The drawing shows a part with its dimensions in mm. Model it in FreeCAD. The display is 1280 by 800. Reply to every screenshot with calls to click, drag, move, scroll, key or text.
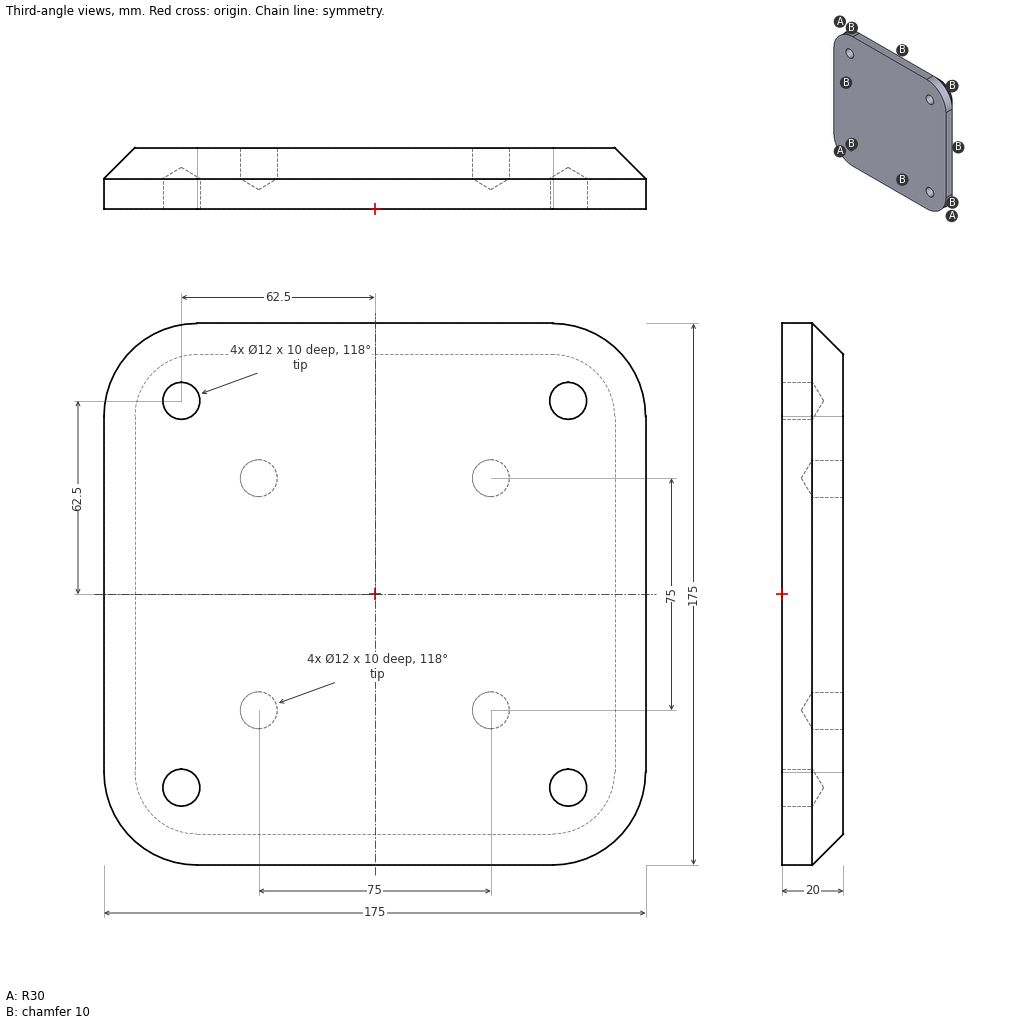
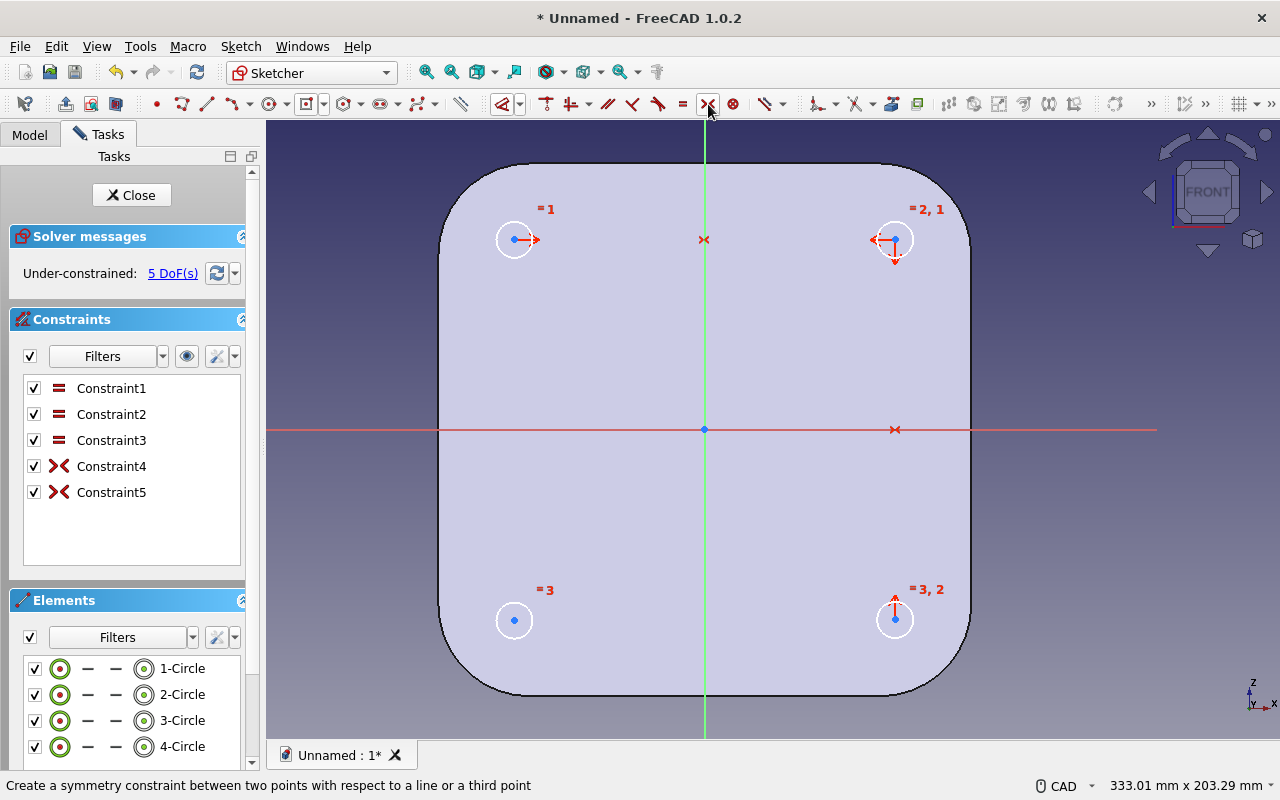
click(514, 240)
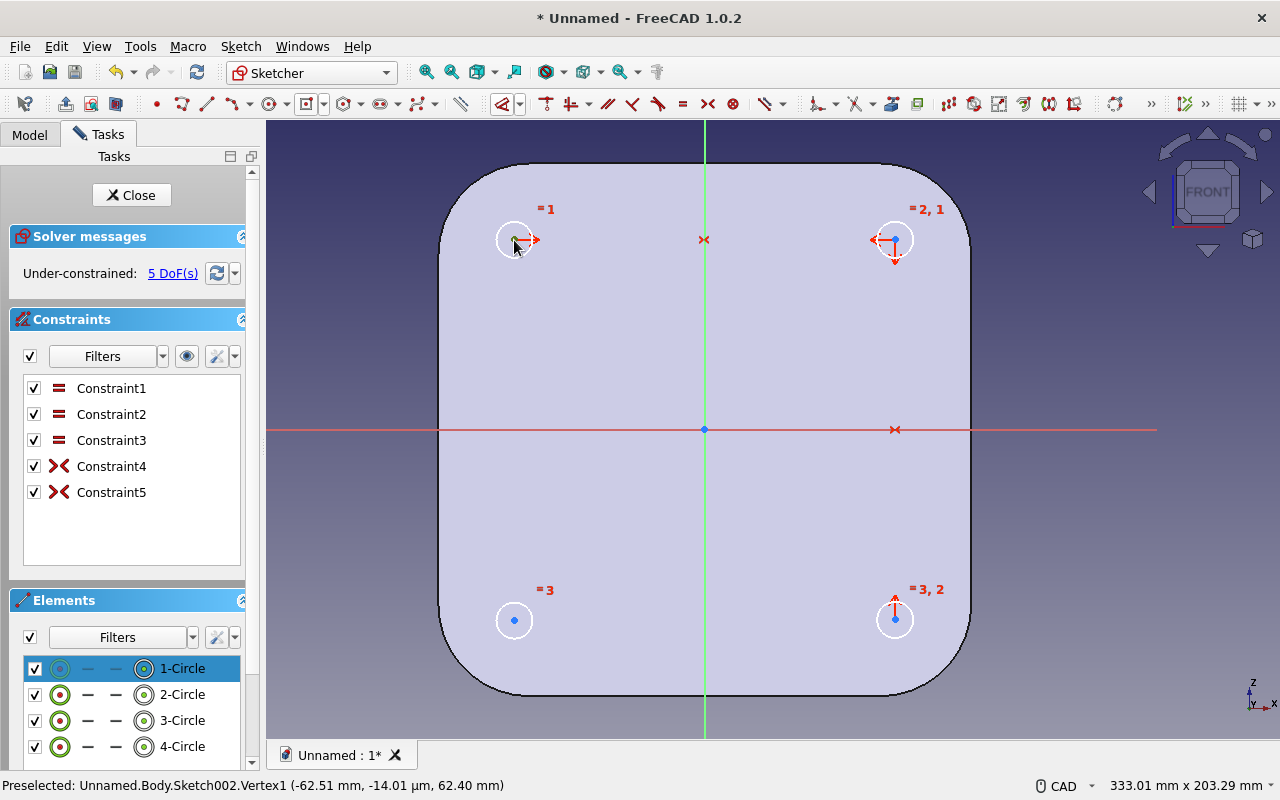
click(514, 621)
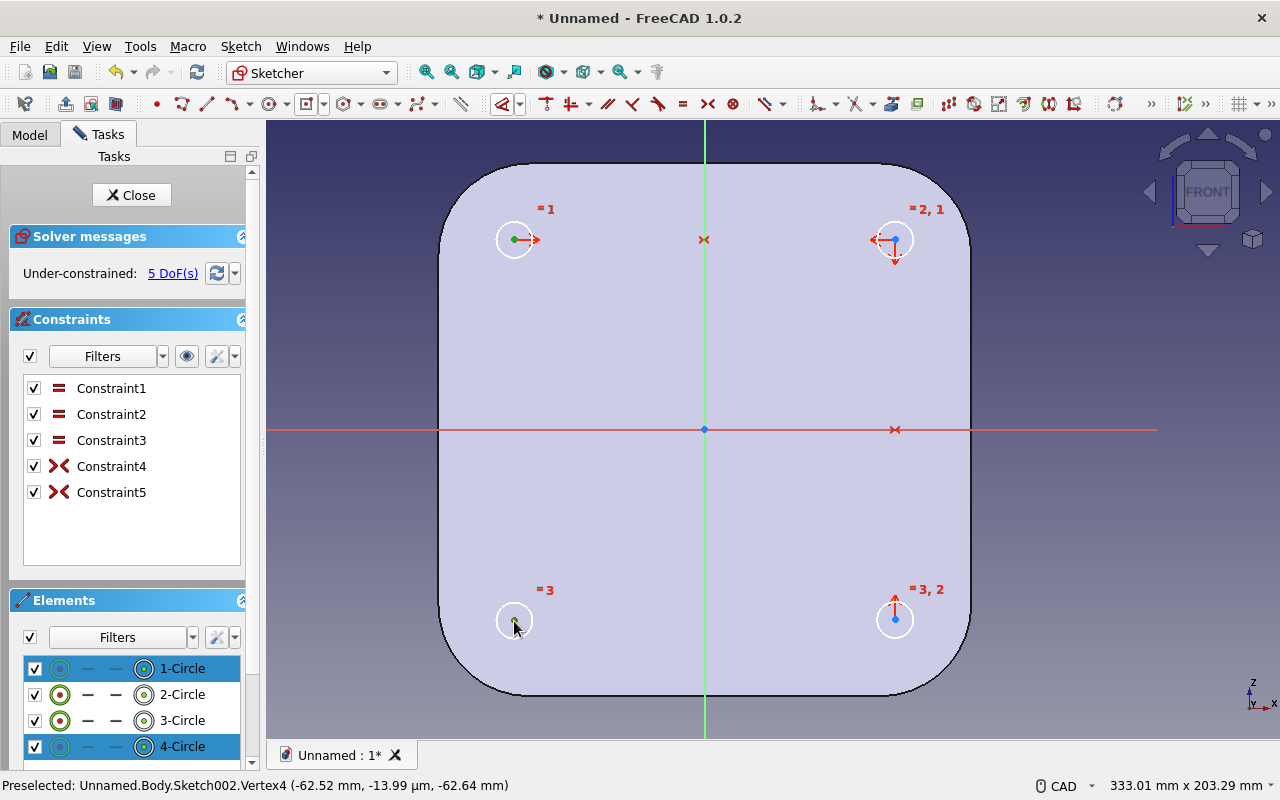
click(353, 430)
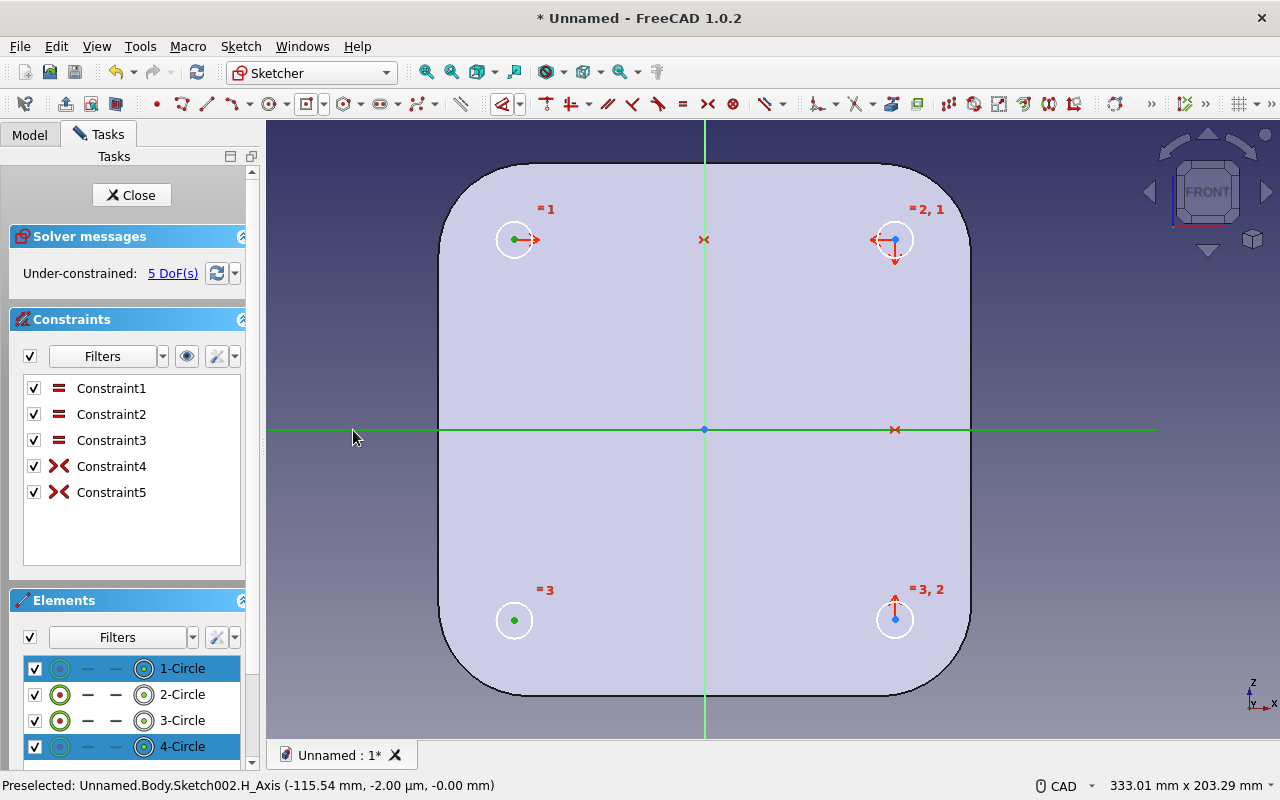
click(708, 104)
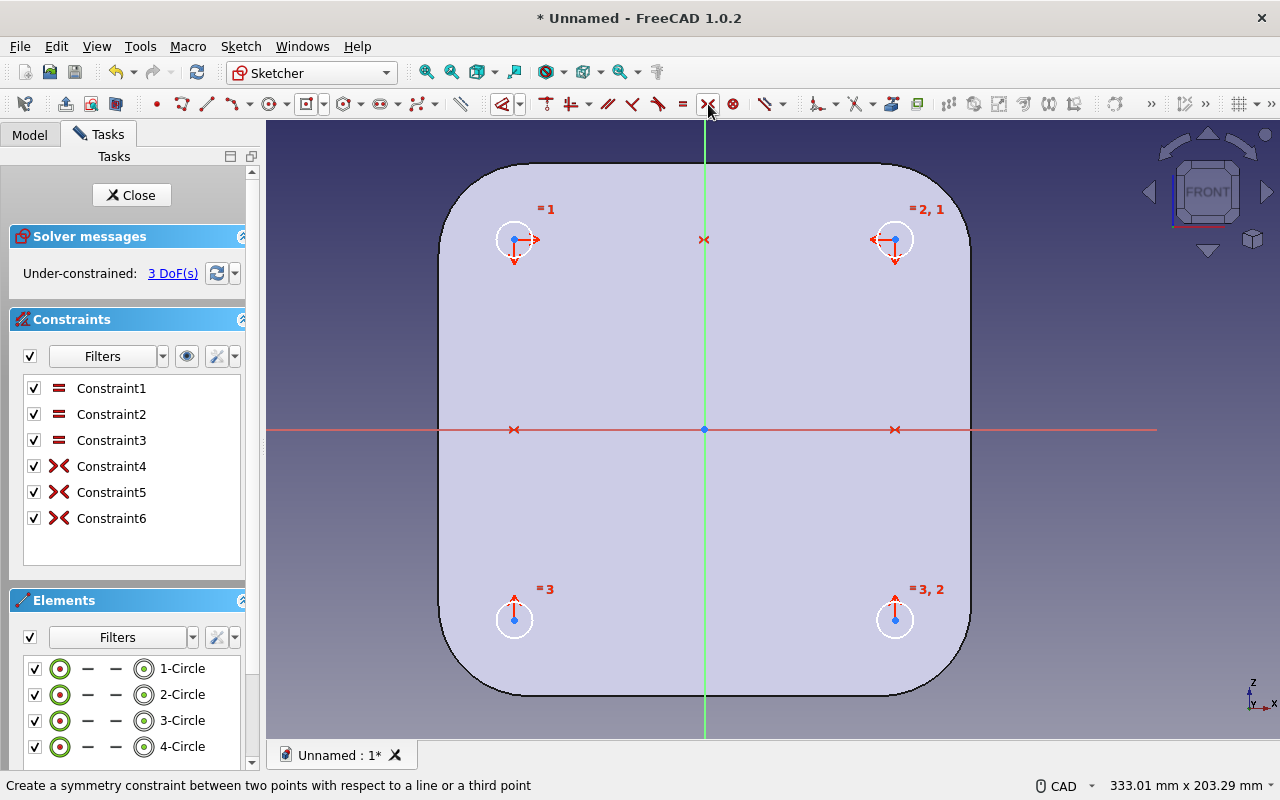
click(527, 227)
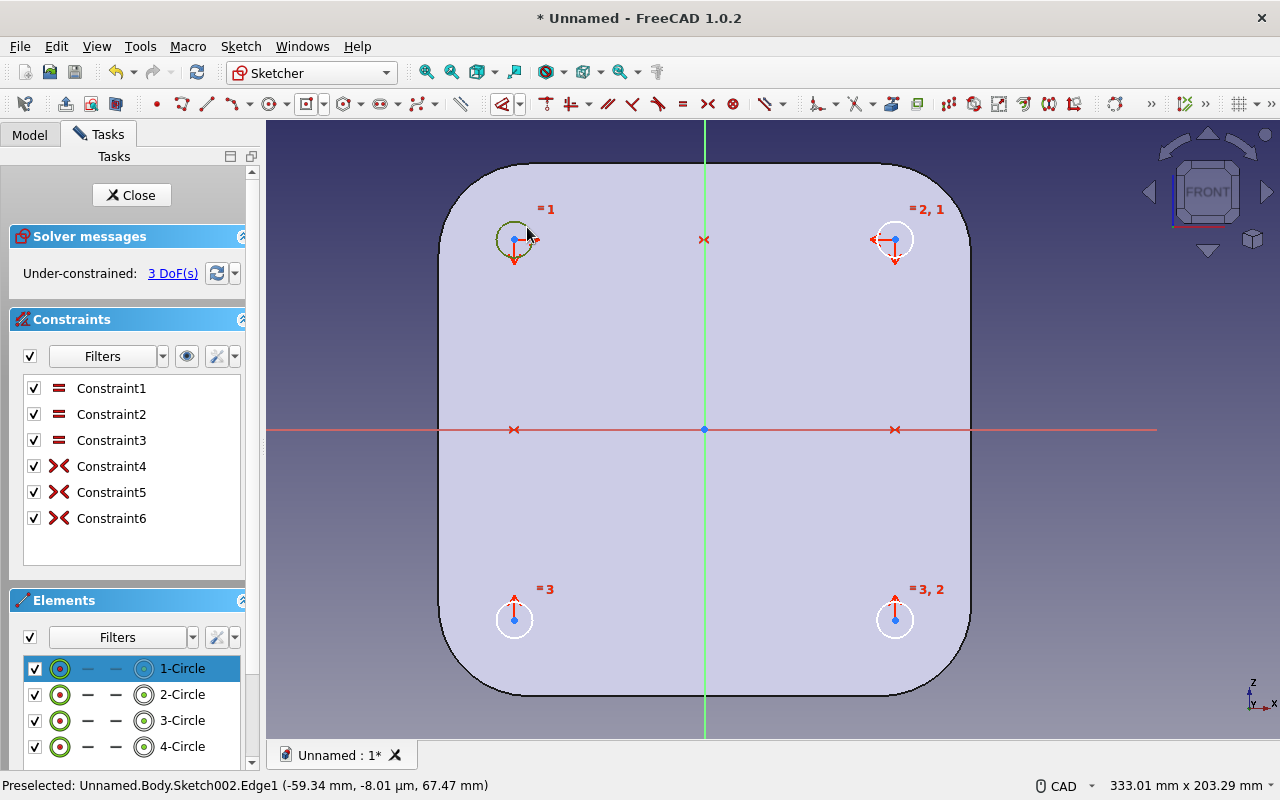
key(k)
key(o)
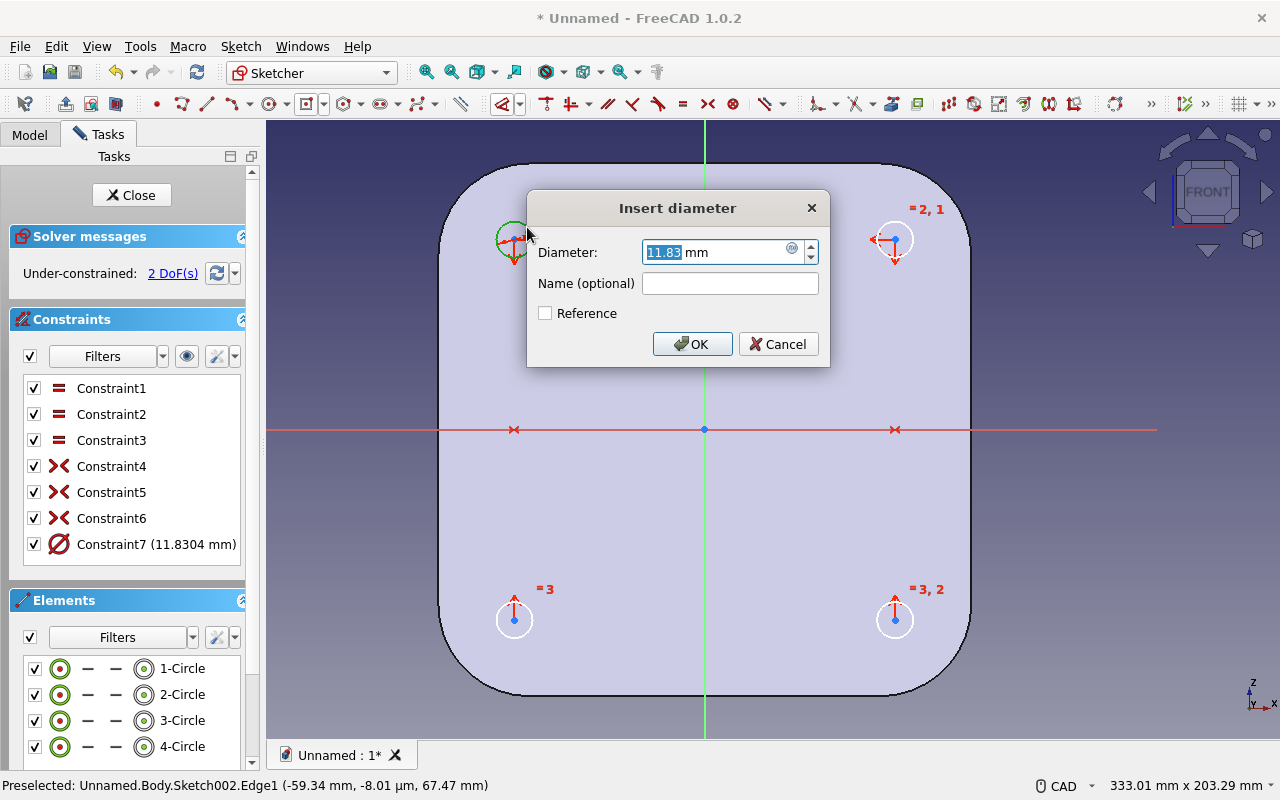
text(12)
key(Return)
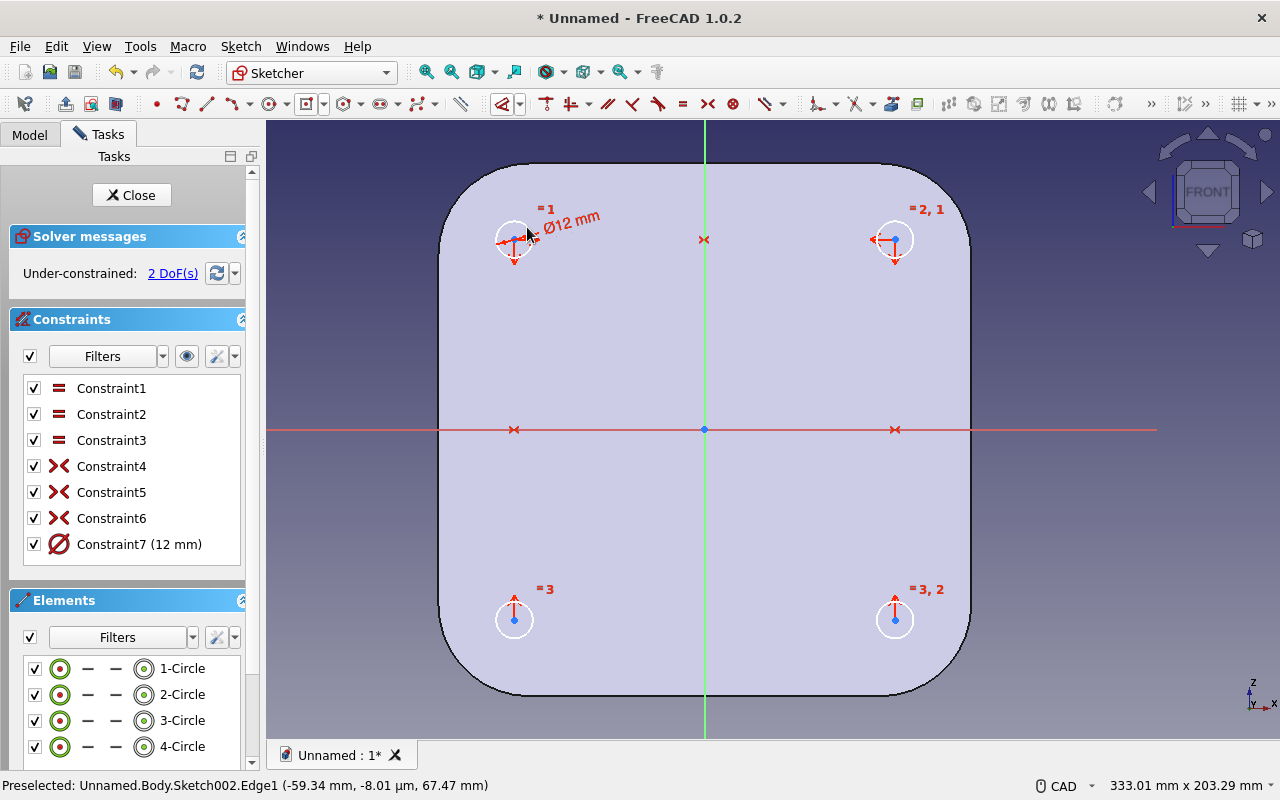
click(514, 240)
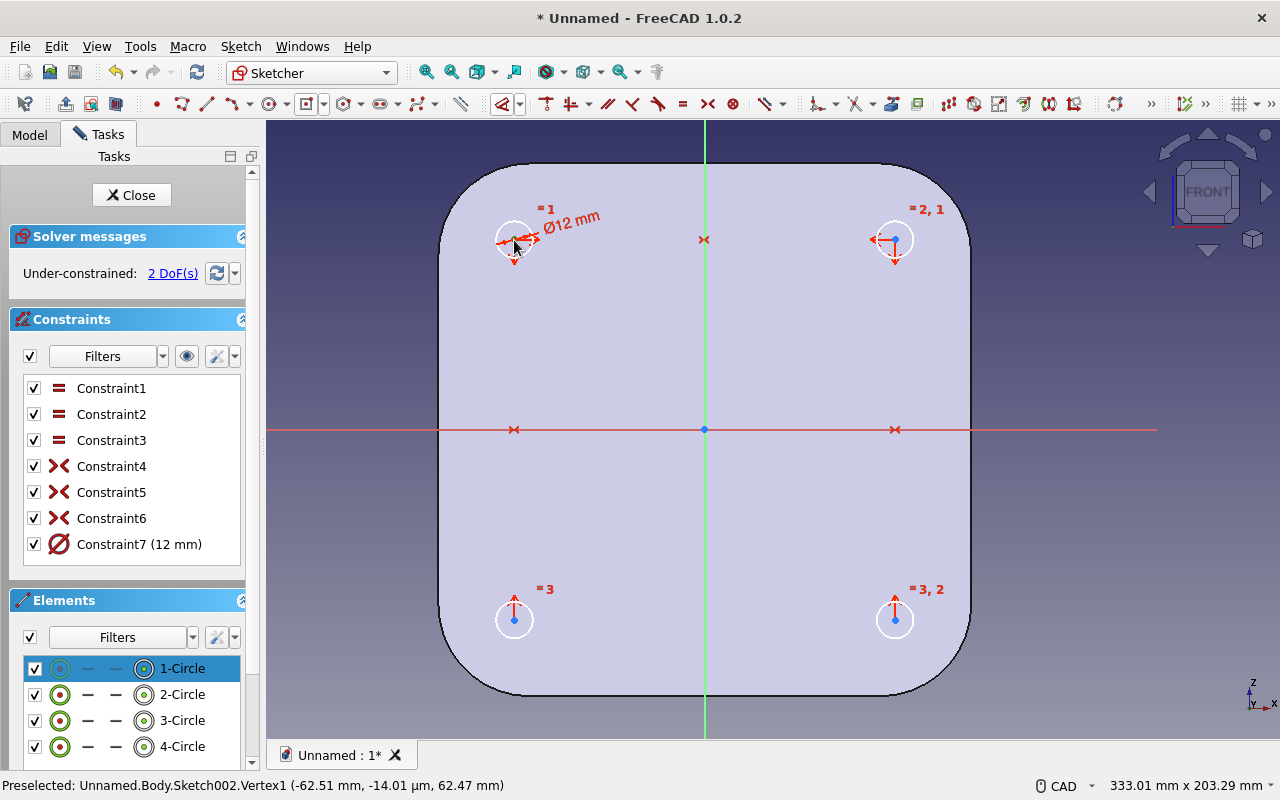
click(520, 104)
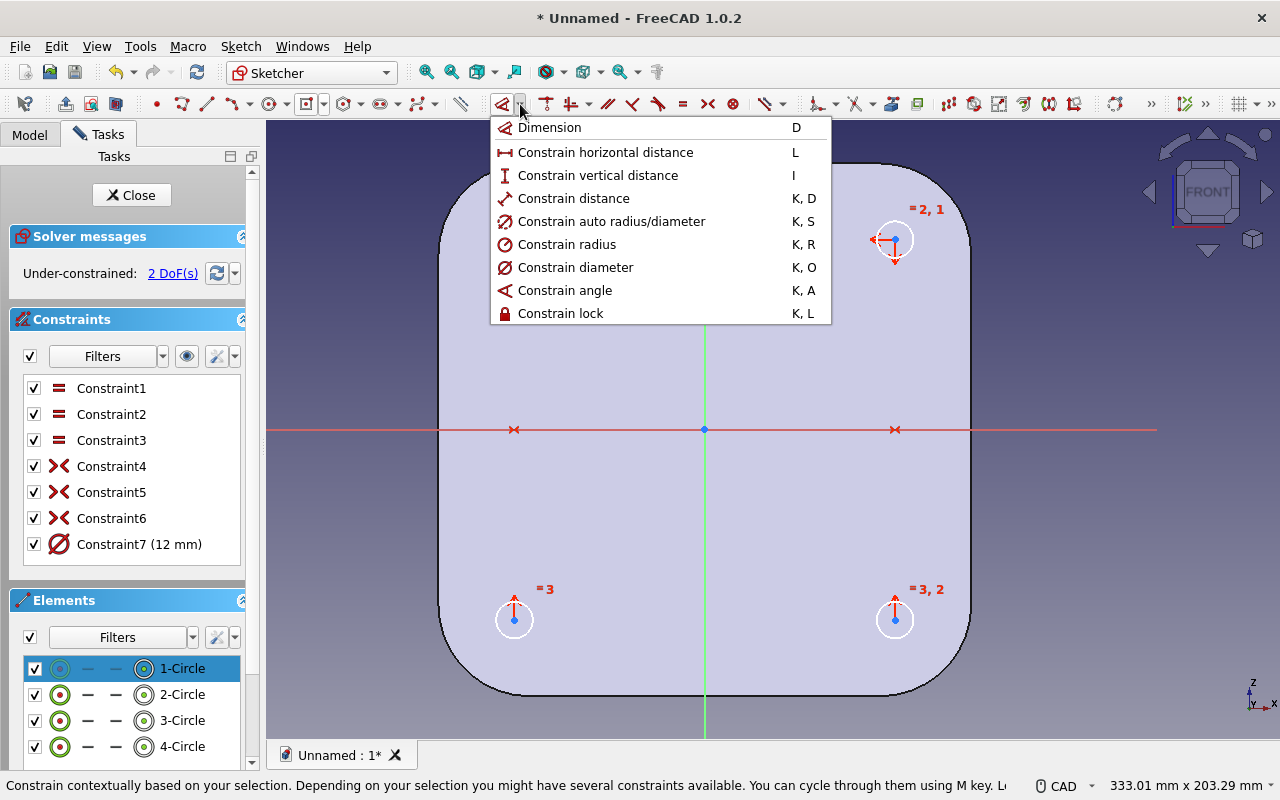
click(661, 152)